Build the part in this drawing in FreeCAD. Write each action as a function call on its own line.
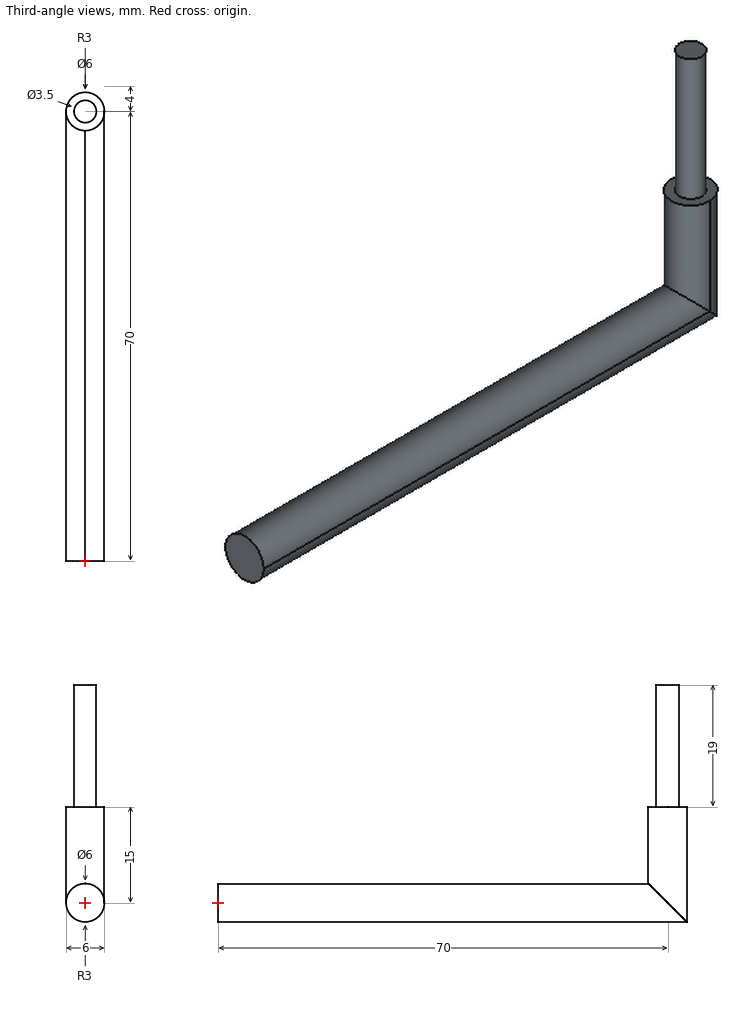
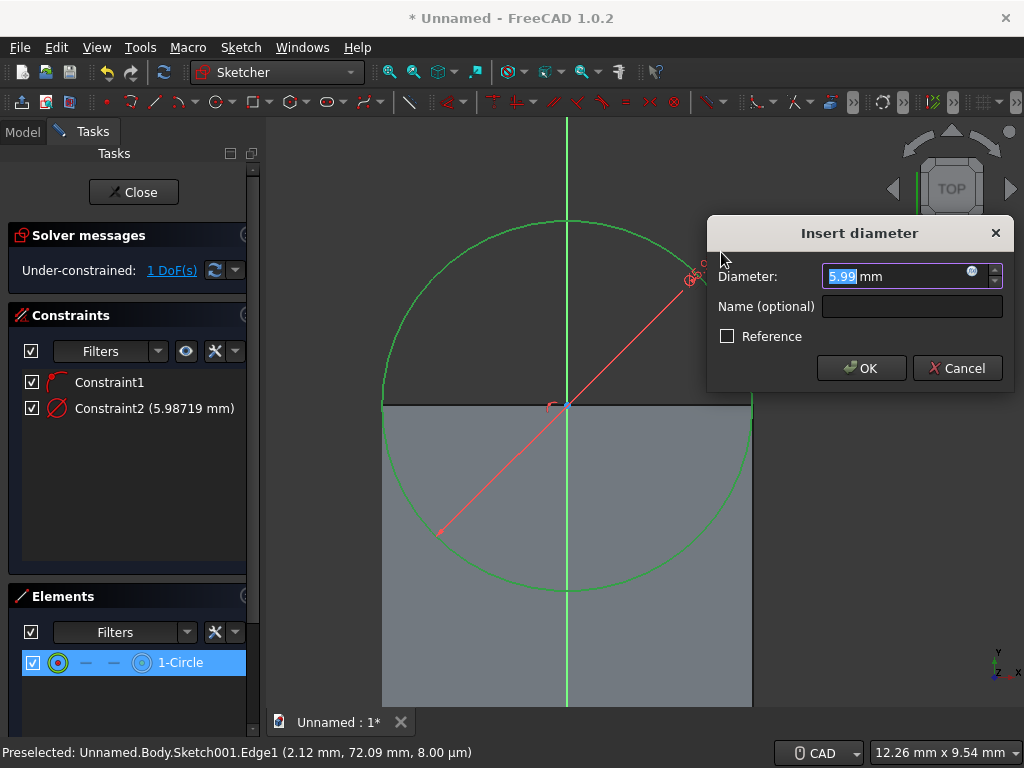
text(6)
key(Return)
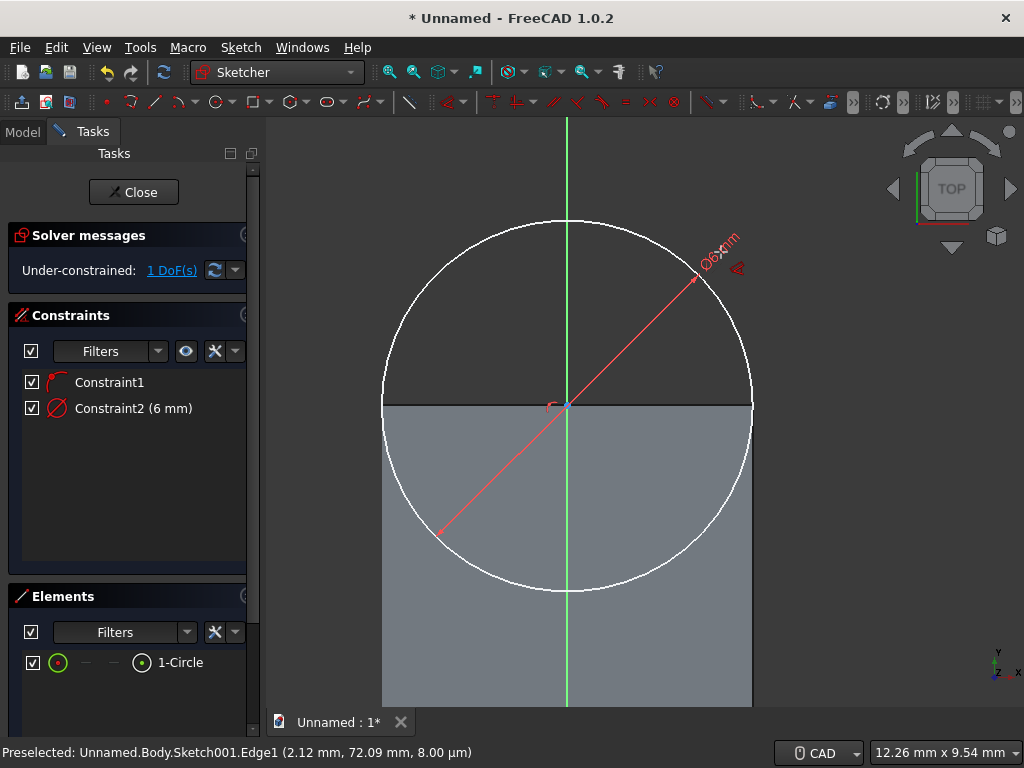
click(567, 406)
click(601, 543)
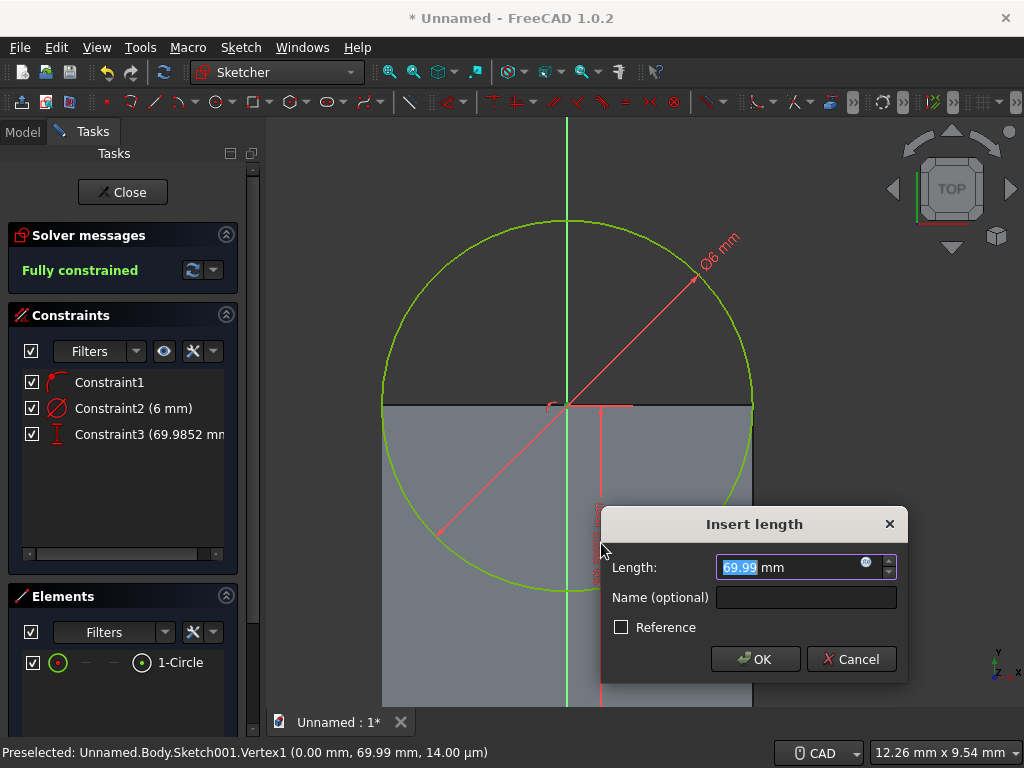
text(70)
key(Return)
key(Escape)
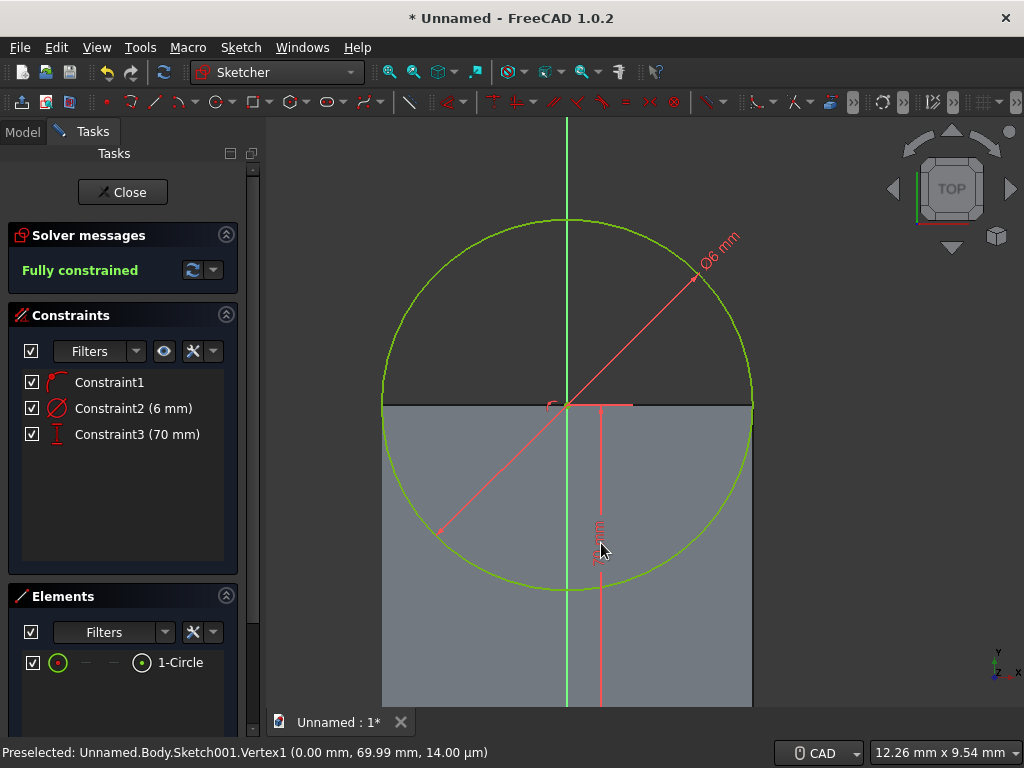
click(123, 192)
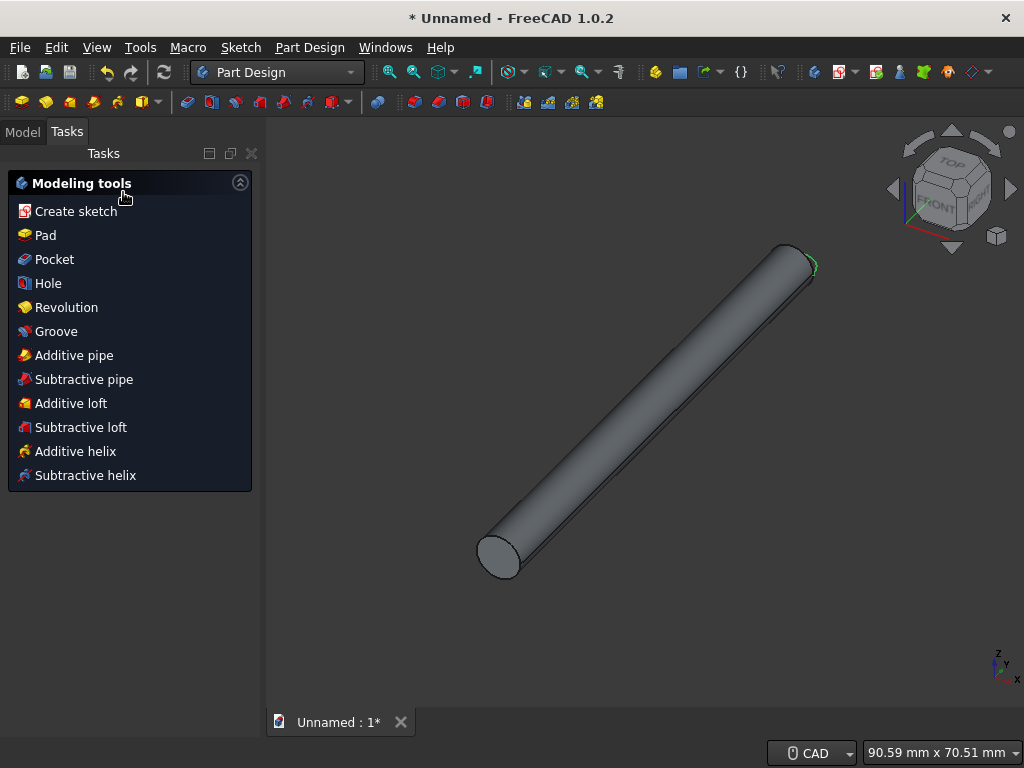
click(22, 102)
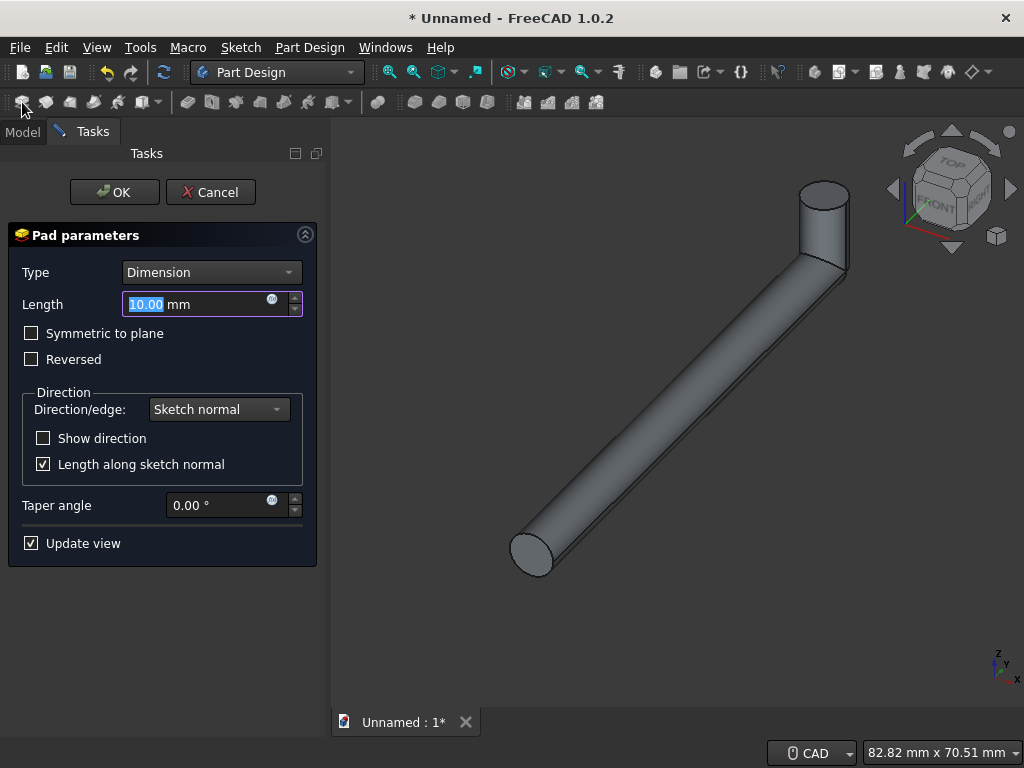
text(15)
key(Tab)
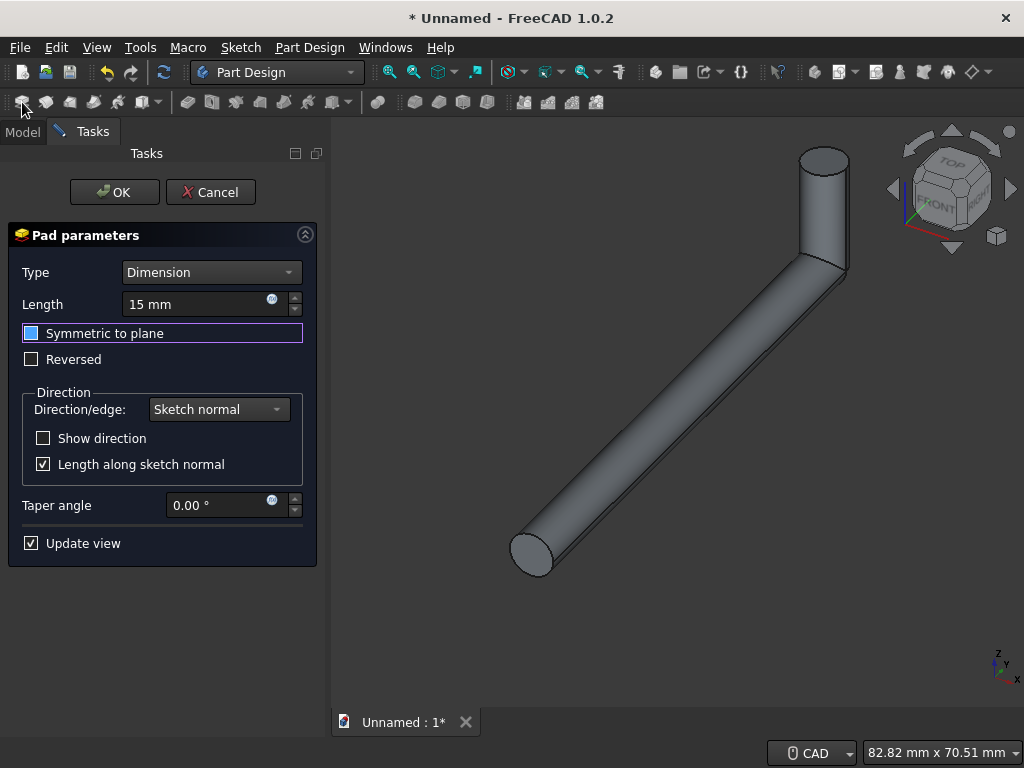
click(115, 192)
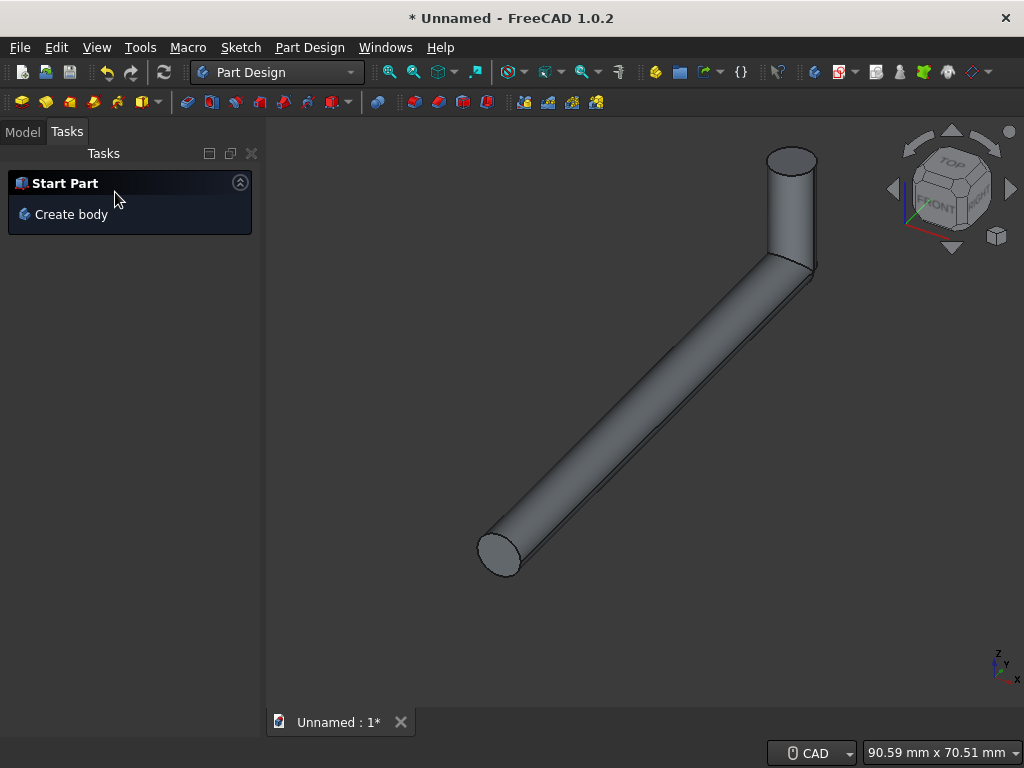
key(4)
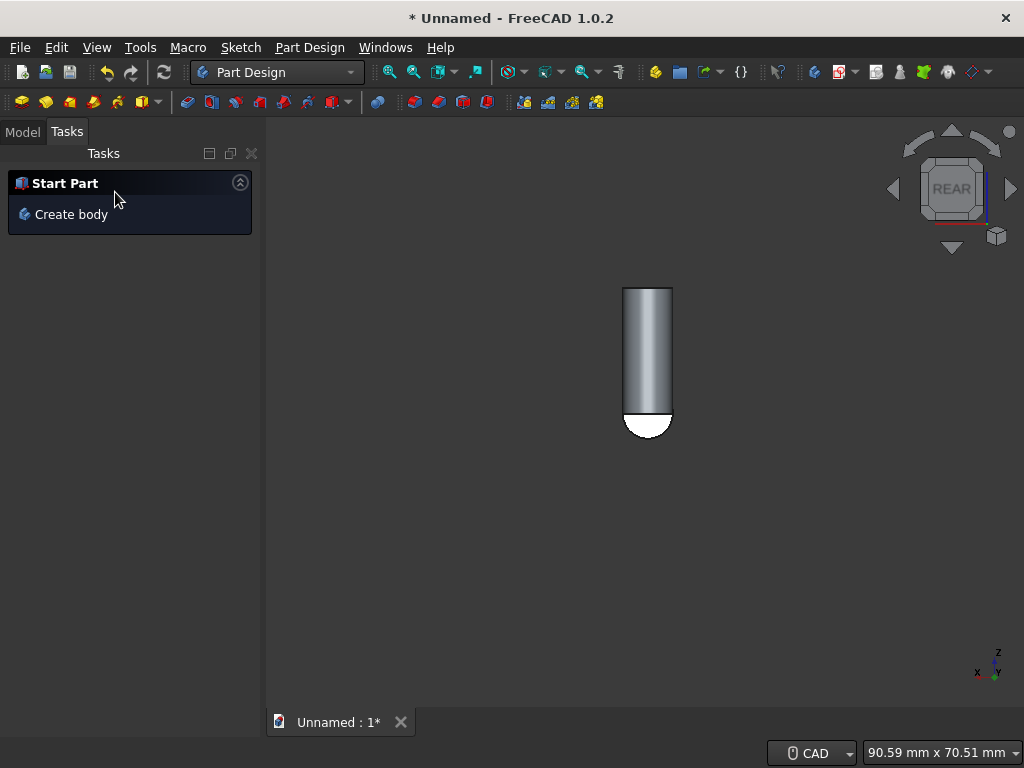
key(v)
key(f)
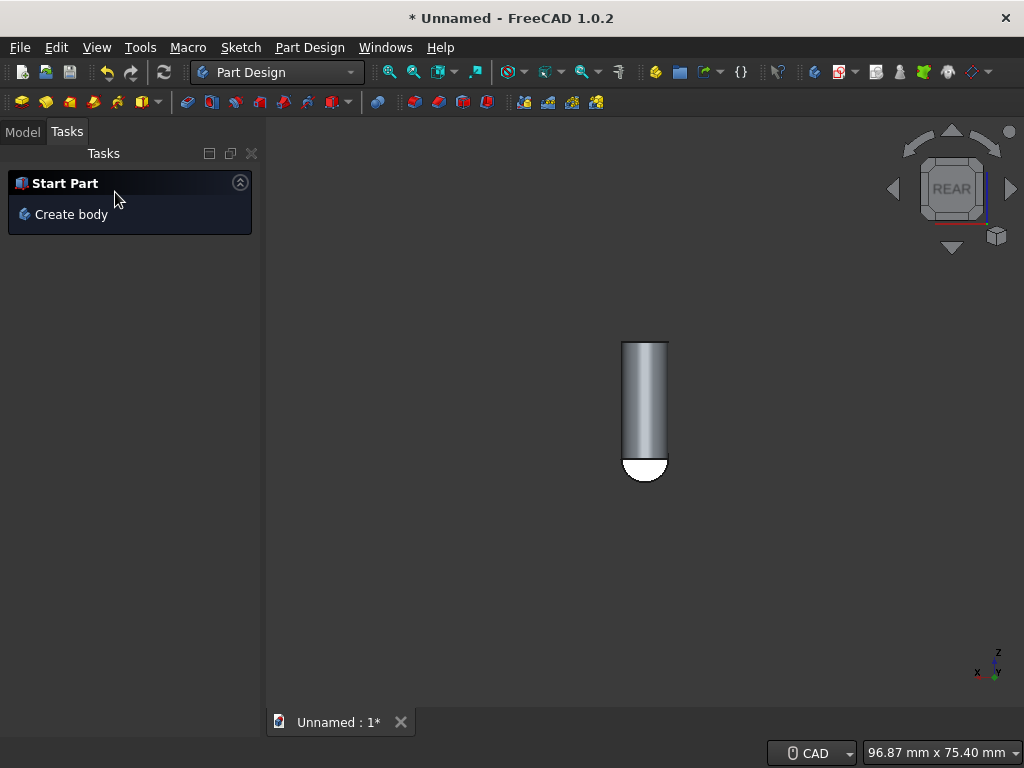
click(645, 470)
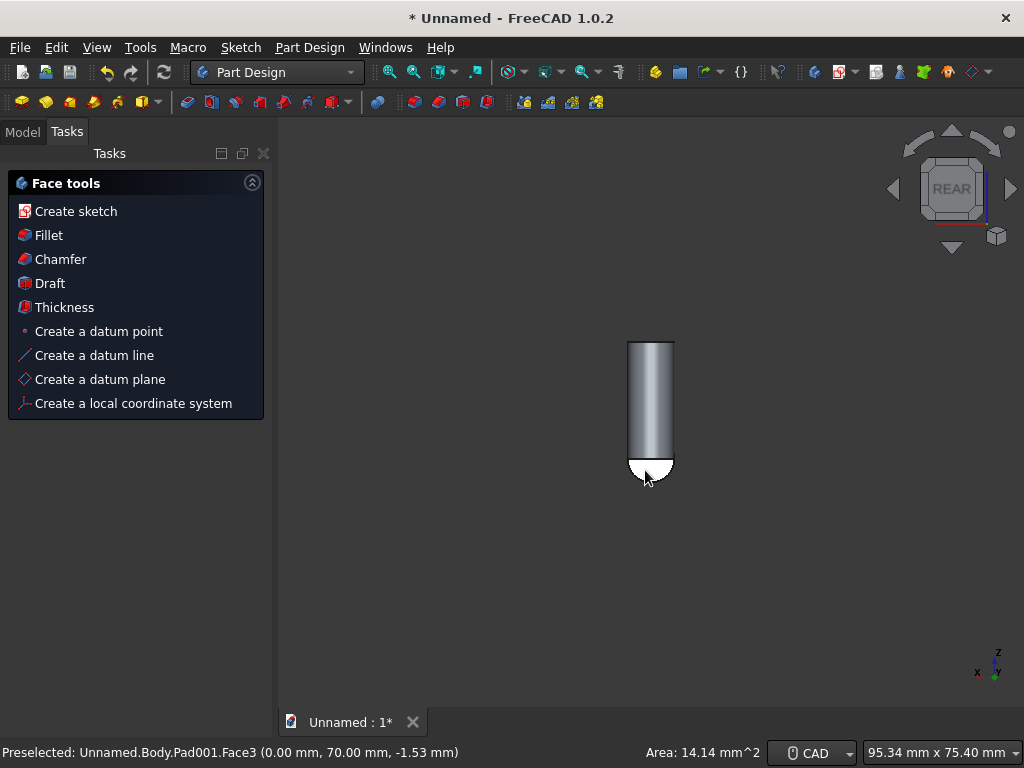
click(840, 72)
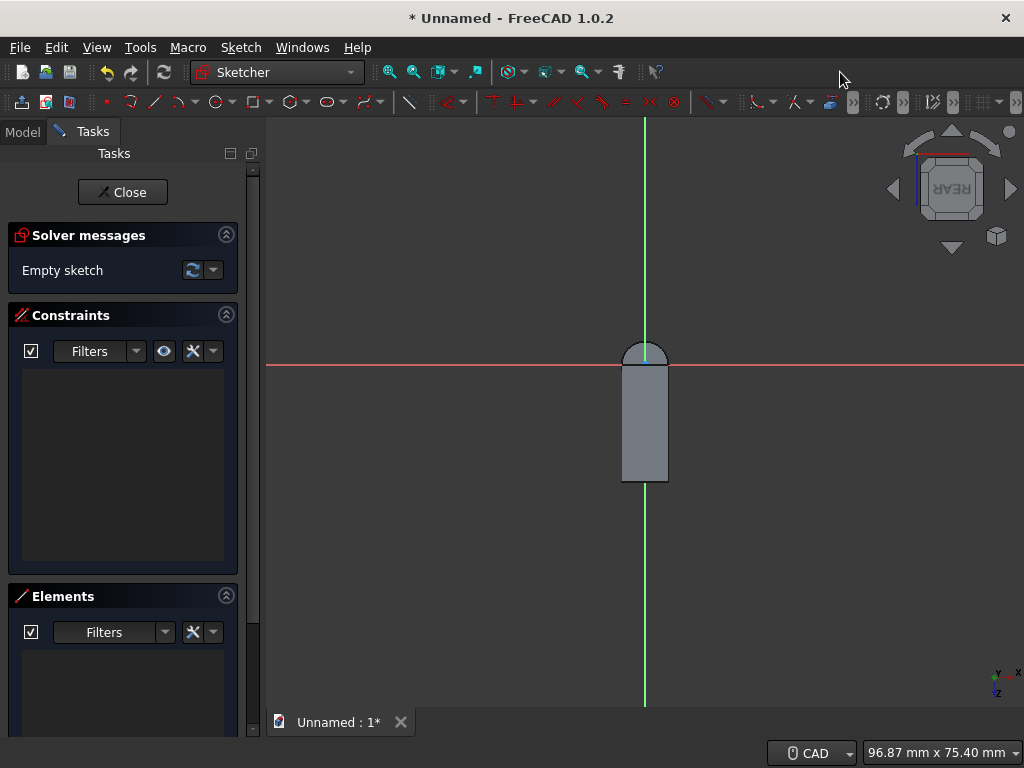
key(q)
key(s)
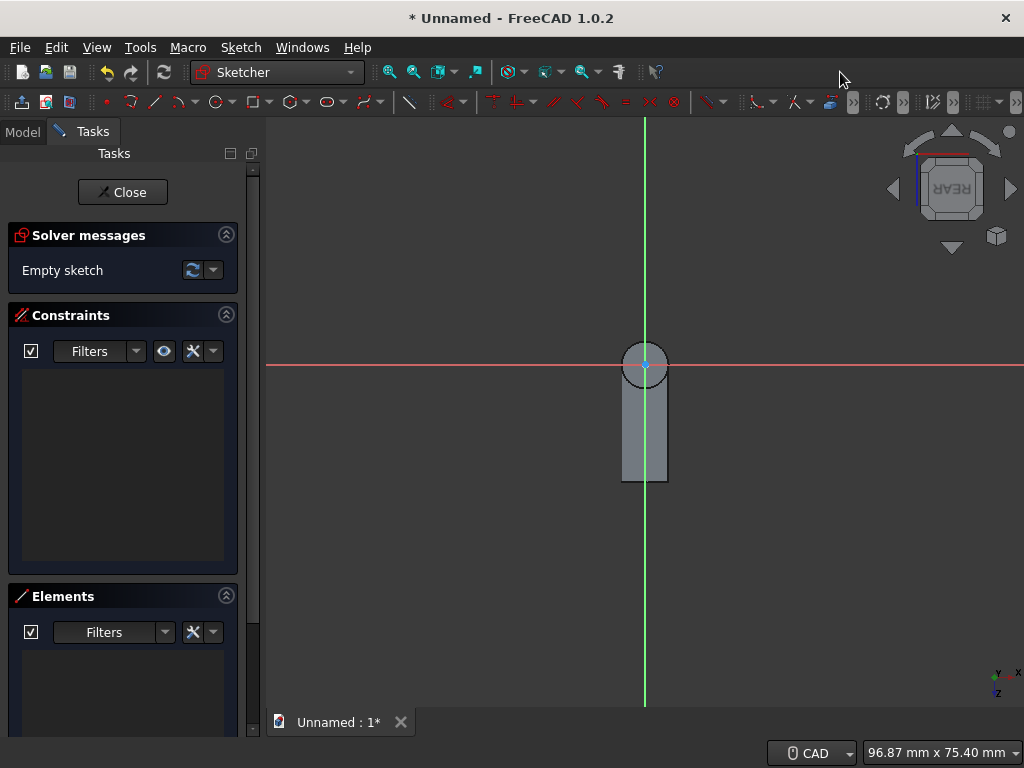
scroll(654, 346, up, 11)